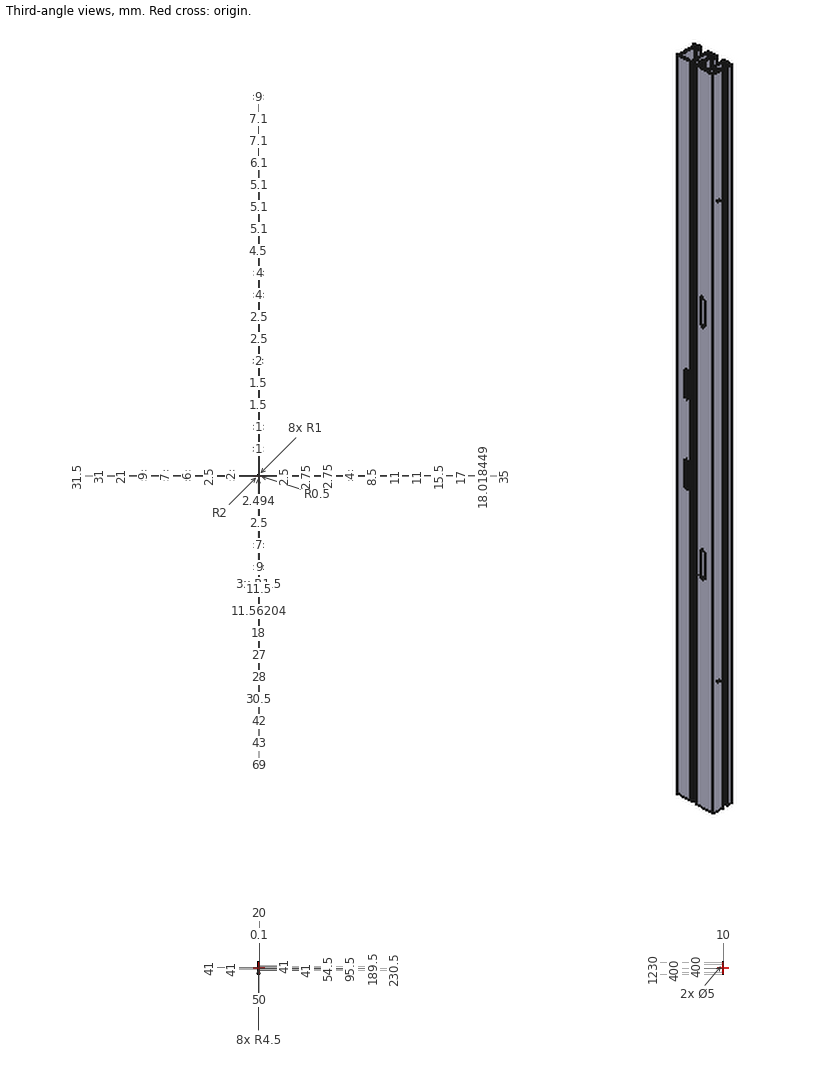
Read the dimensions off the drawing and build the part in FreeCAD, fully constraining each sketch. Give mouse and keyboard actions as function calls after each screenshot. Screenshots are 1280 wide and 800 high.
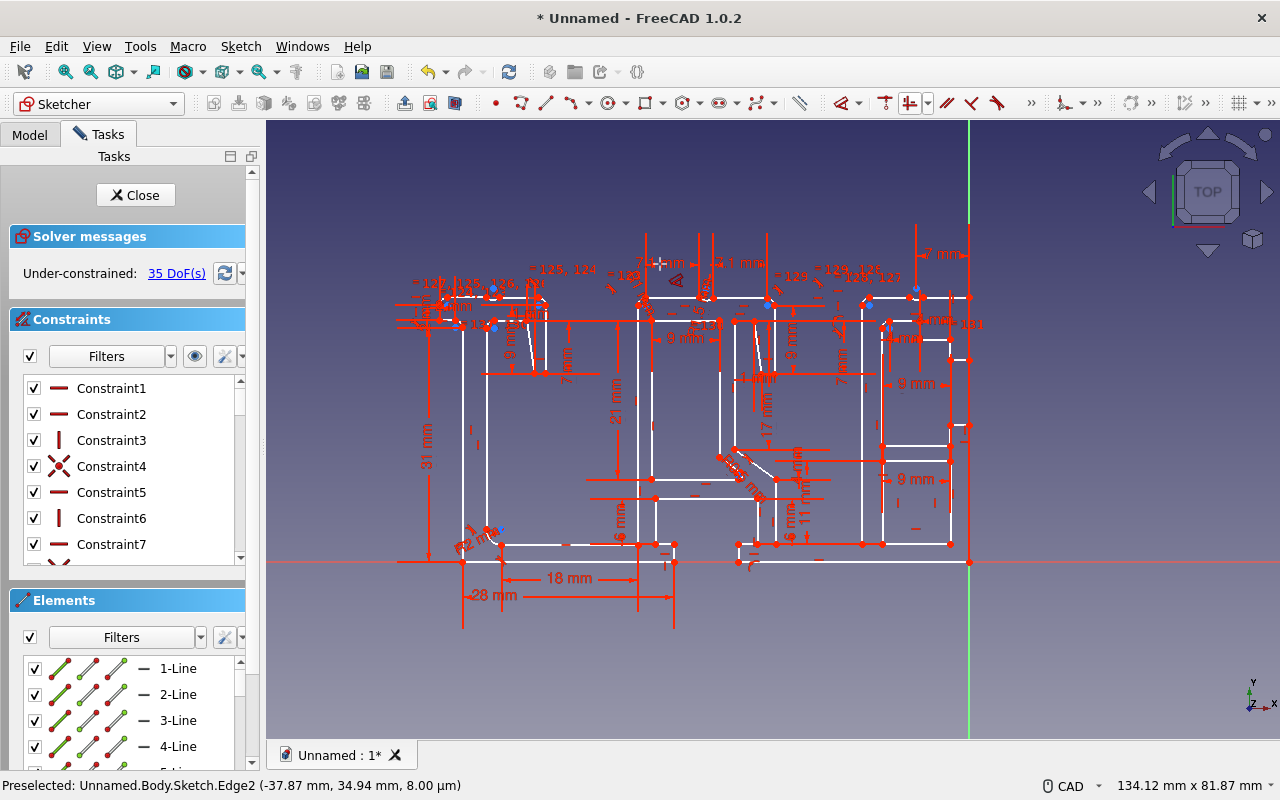
scroll(504, 321, up, 2)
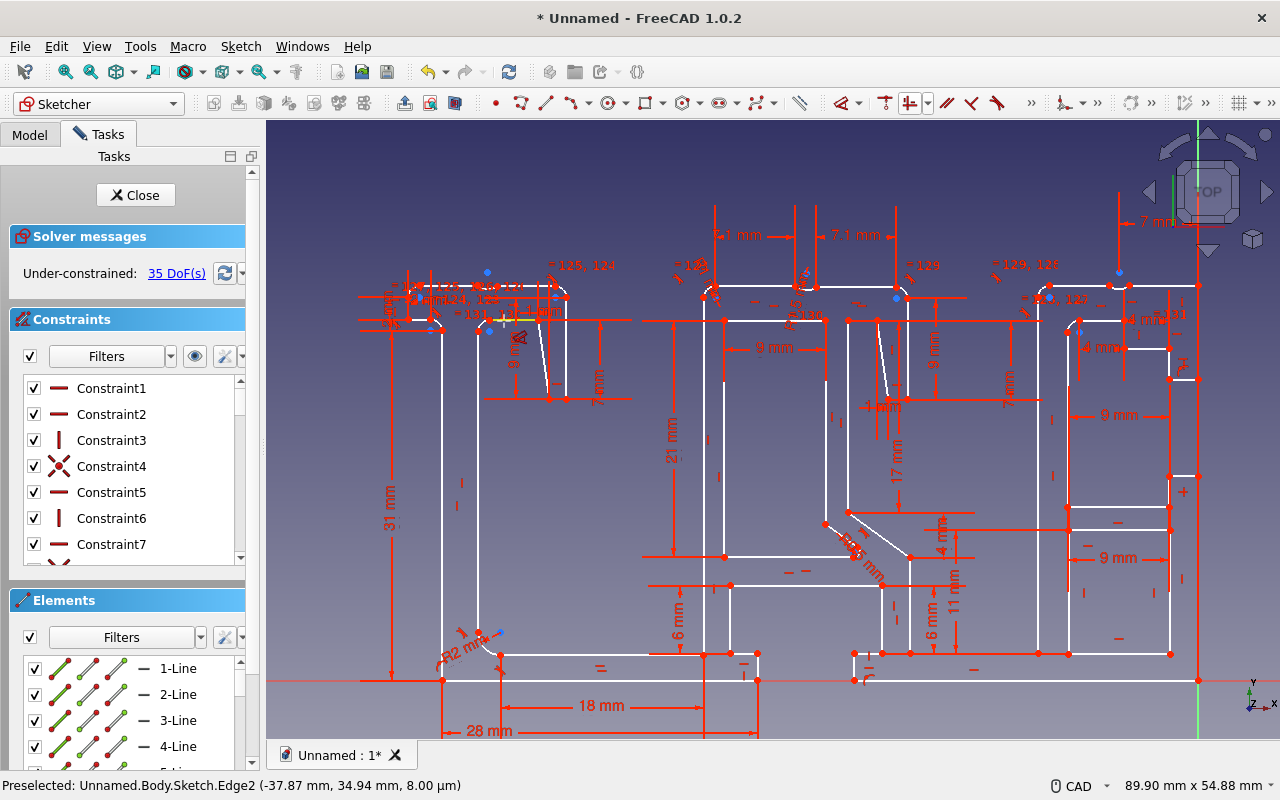
click(504, 320)
click(514, 262)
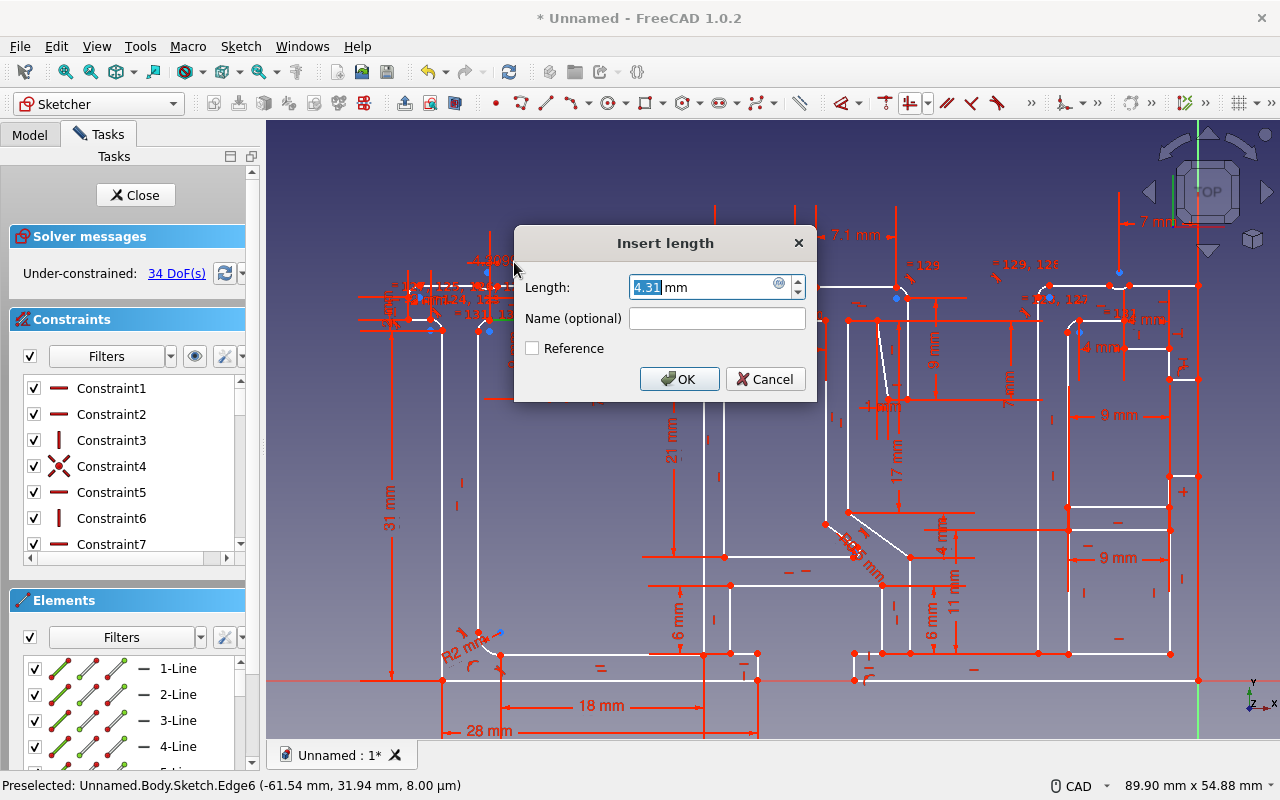
text(4.5)
key(Return)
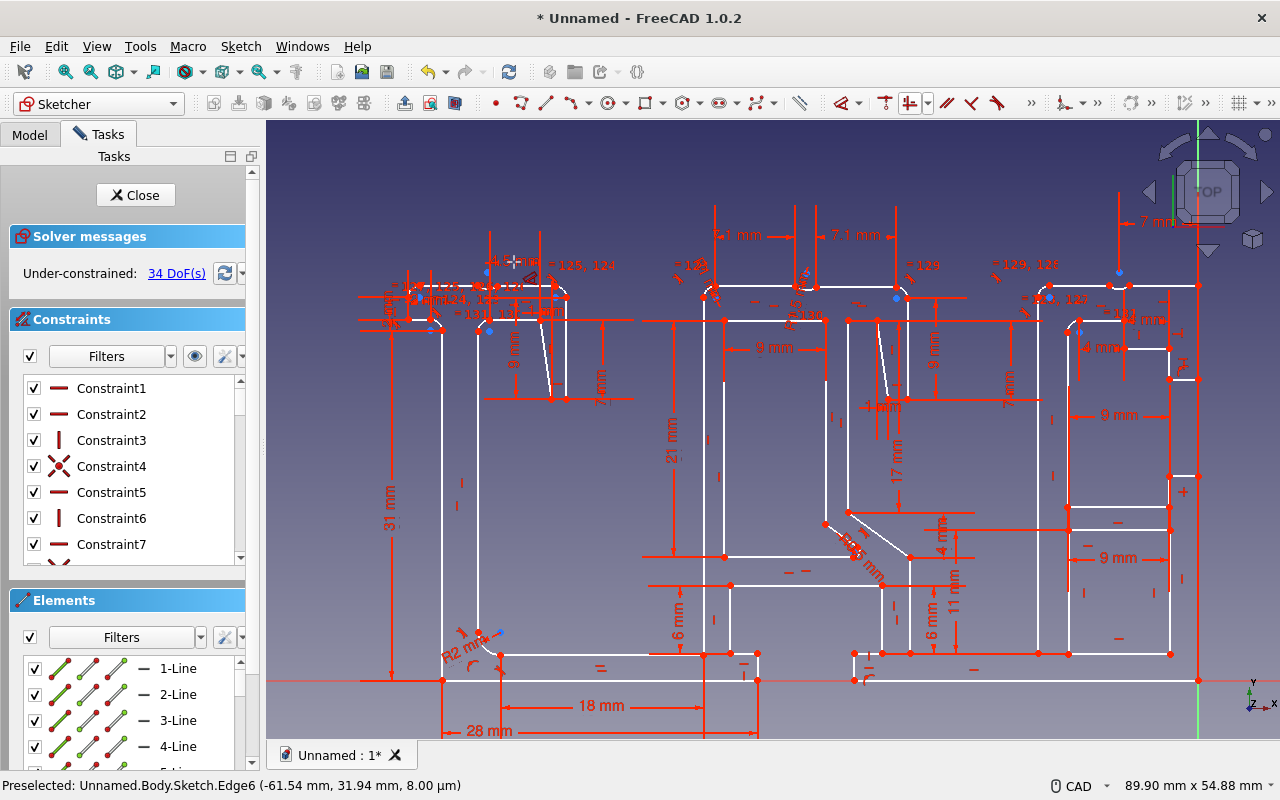
scroll(559, 399, up, 5)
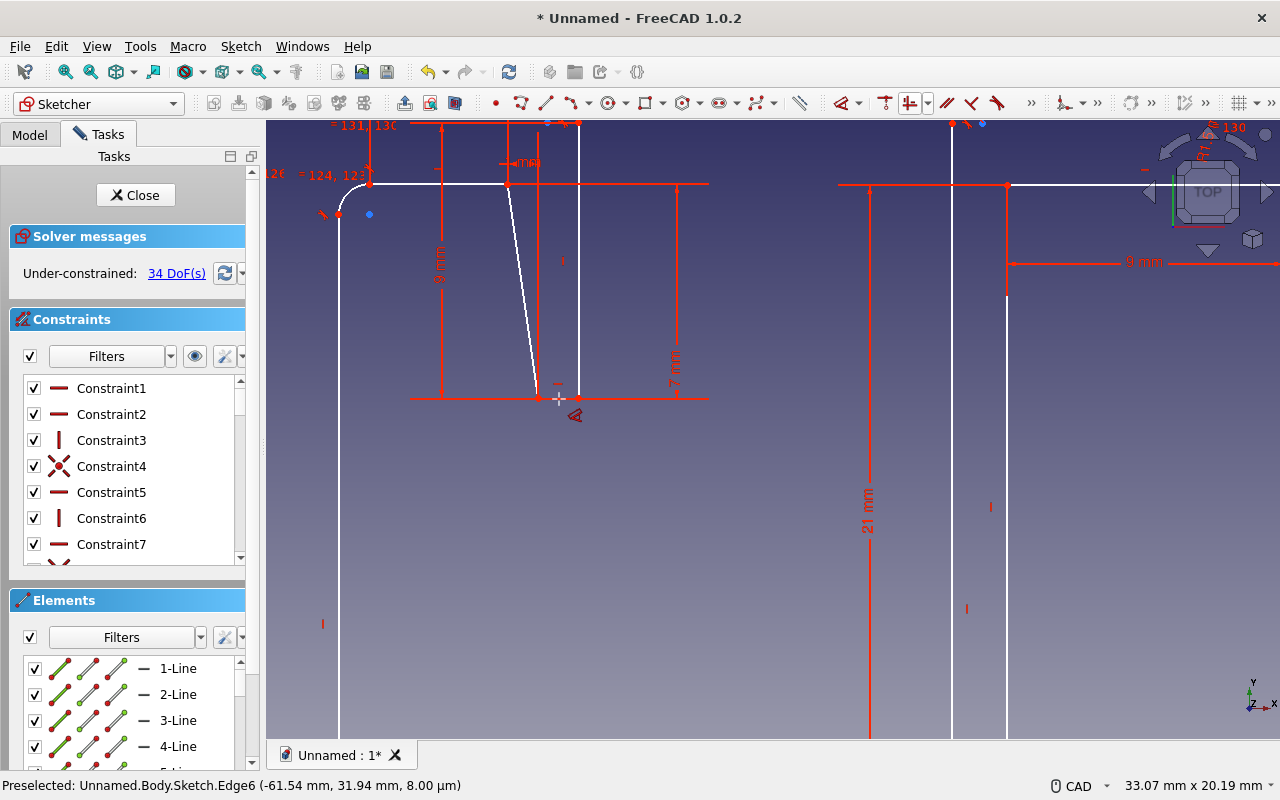
click(558, 399)
click(558, 365)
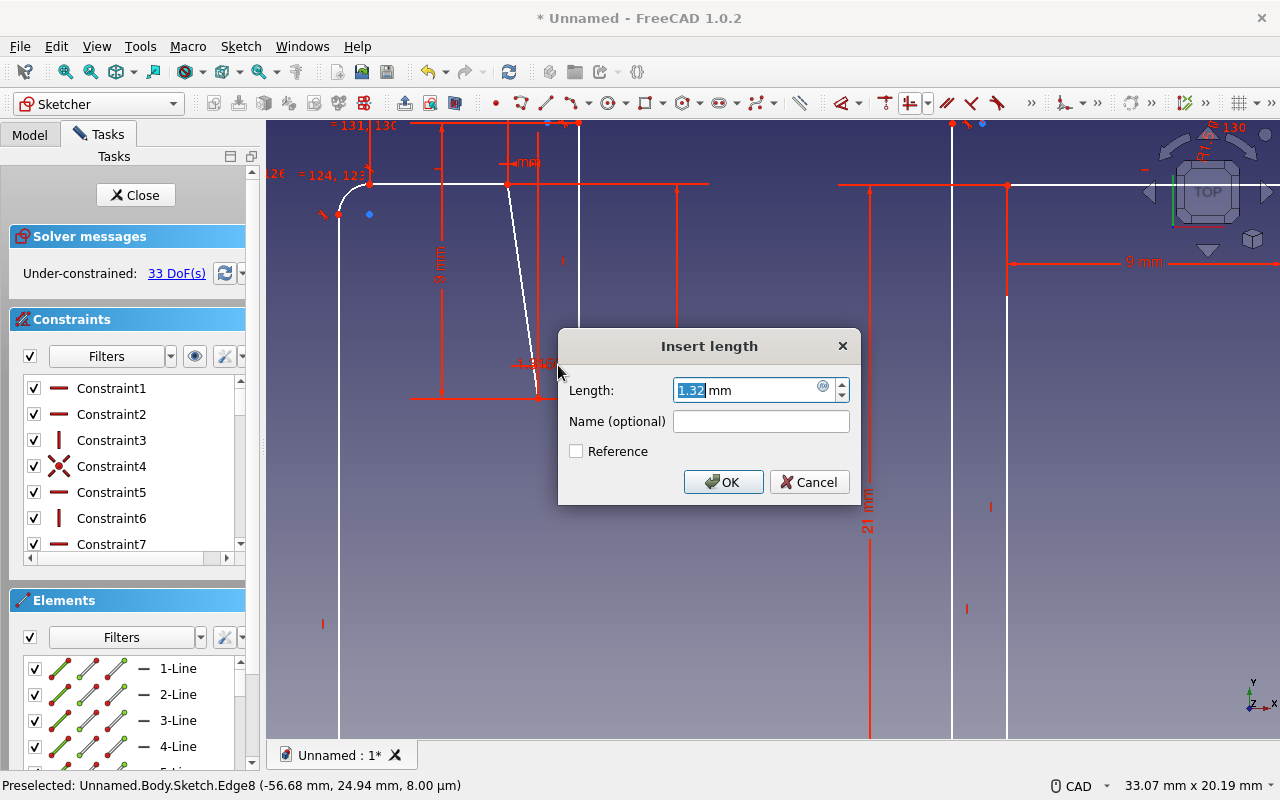
text(1.5)
key(Return)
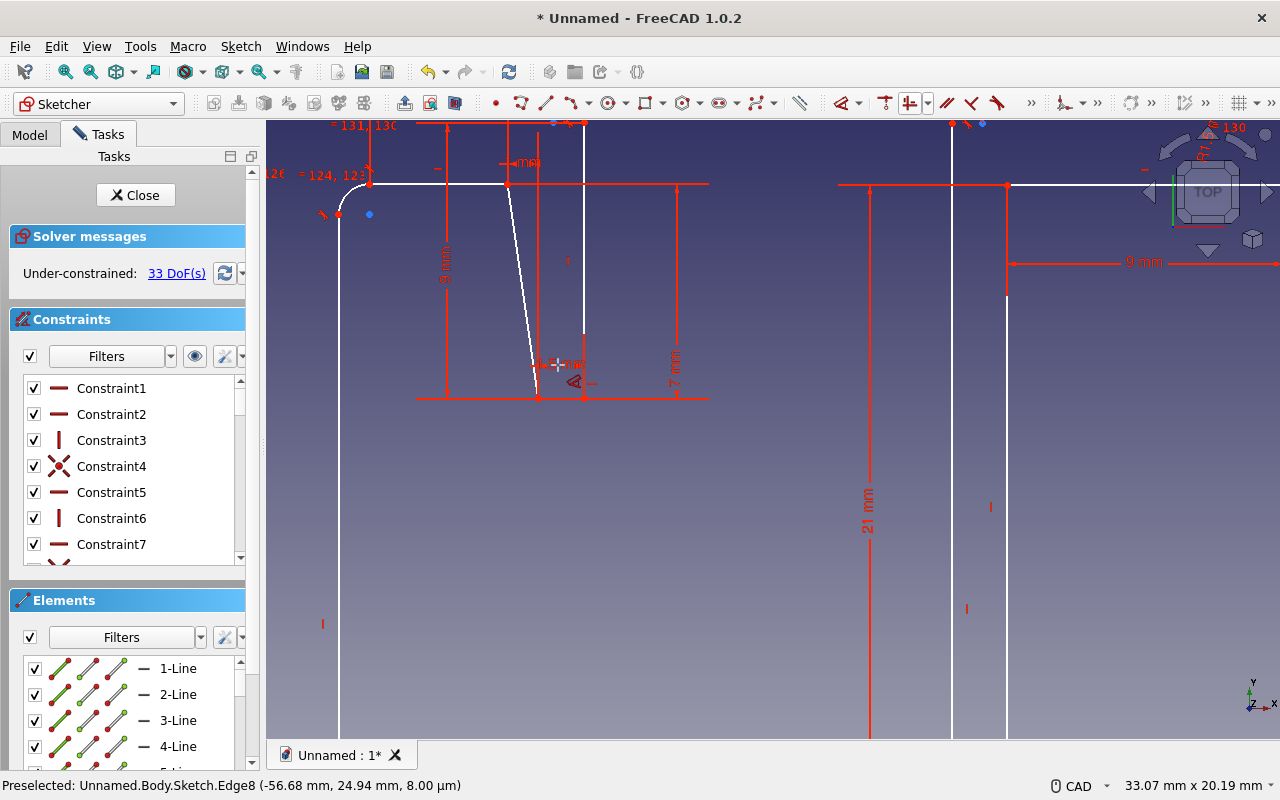
scroll(535, 365, down, 7)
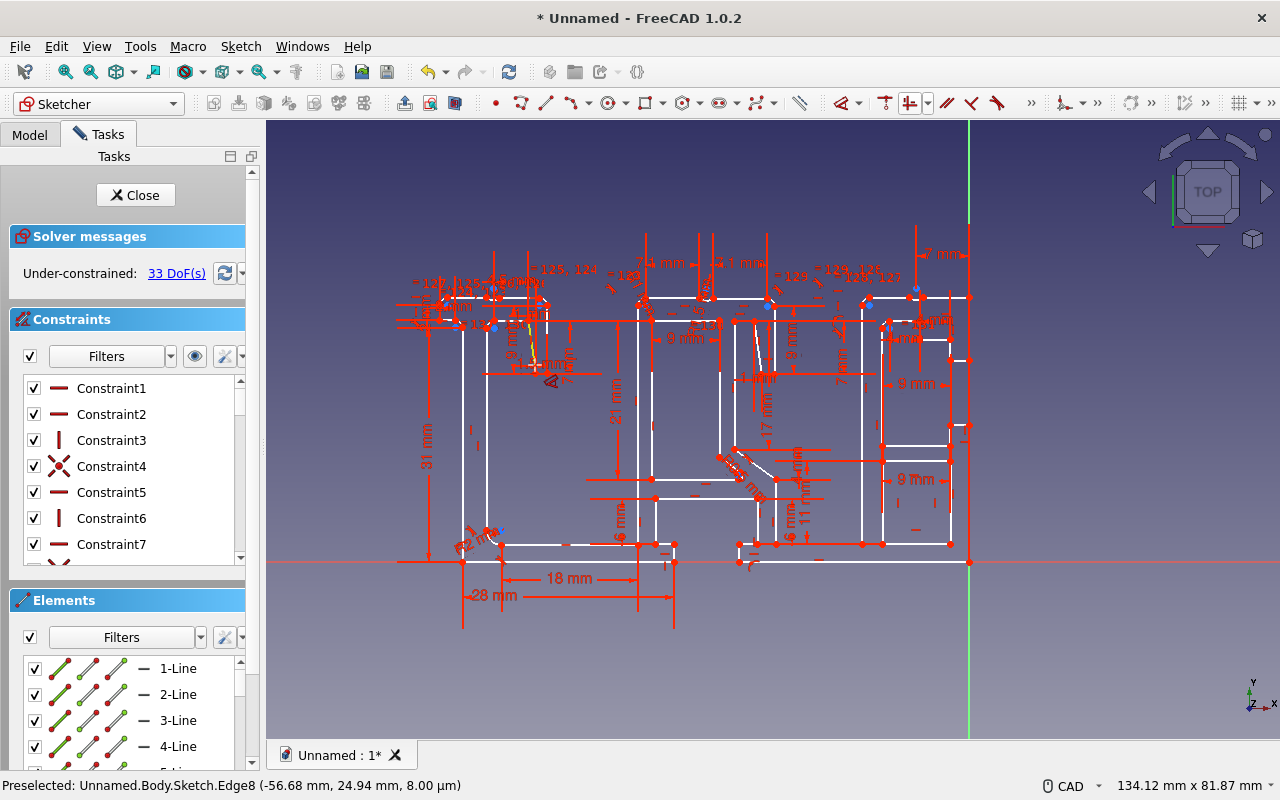
click(528, 298)
click(520, 240)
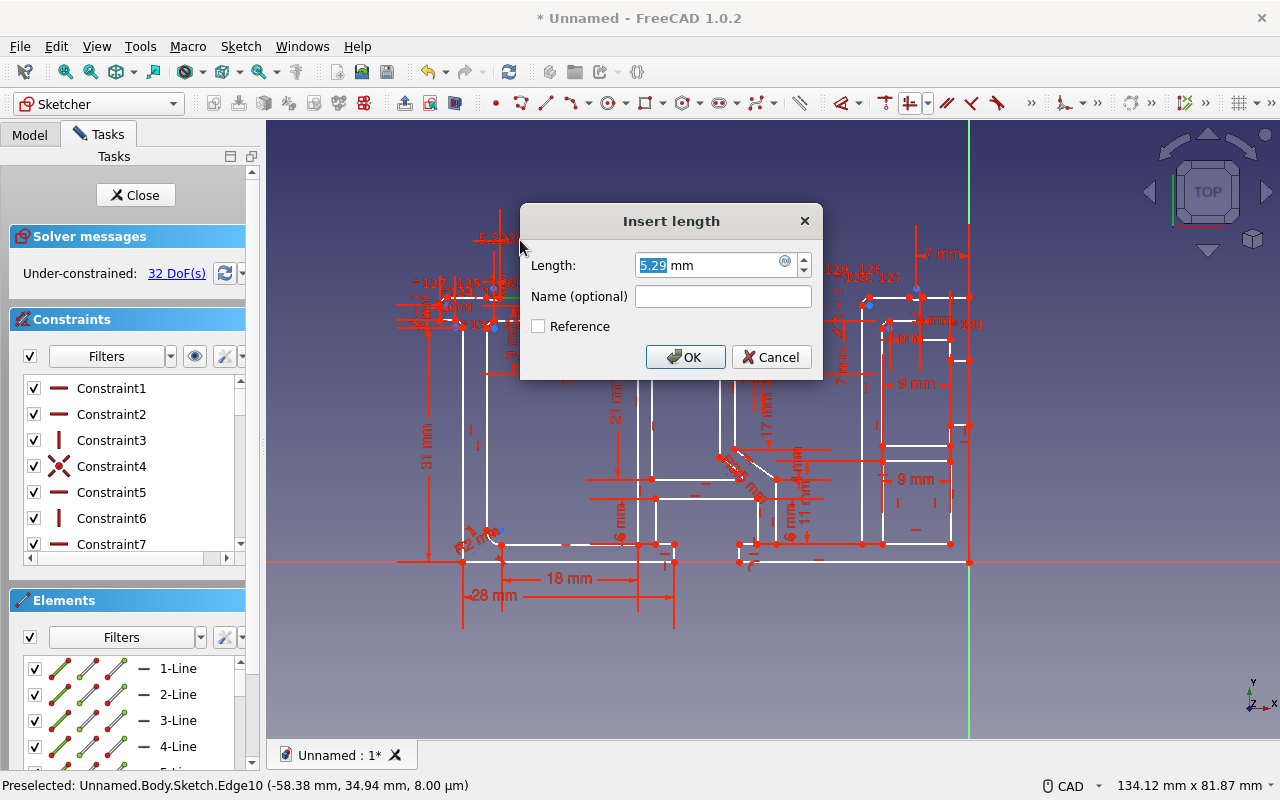
text(5.1)
key(Return)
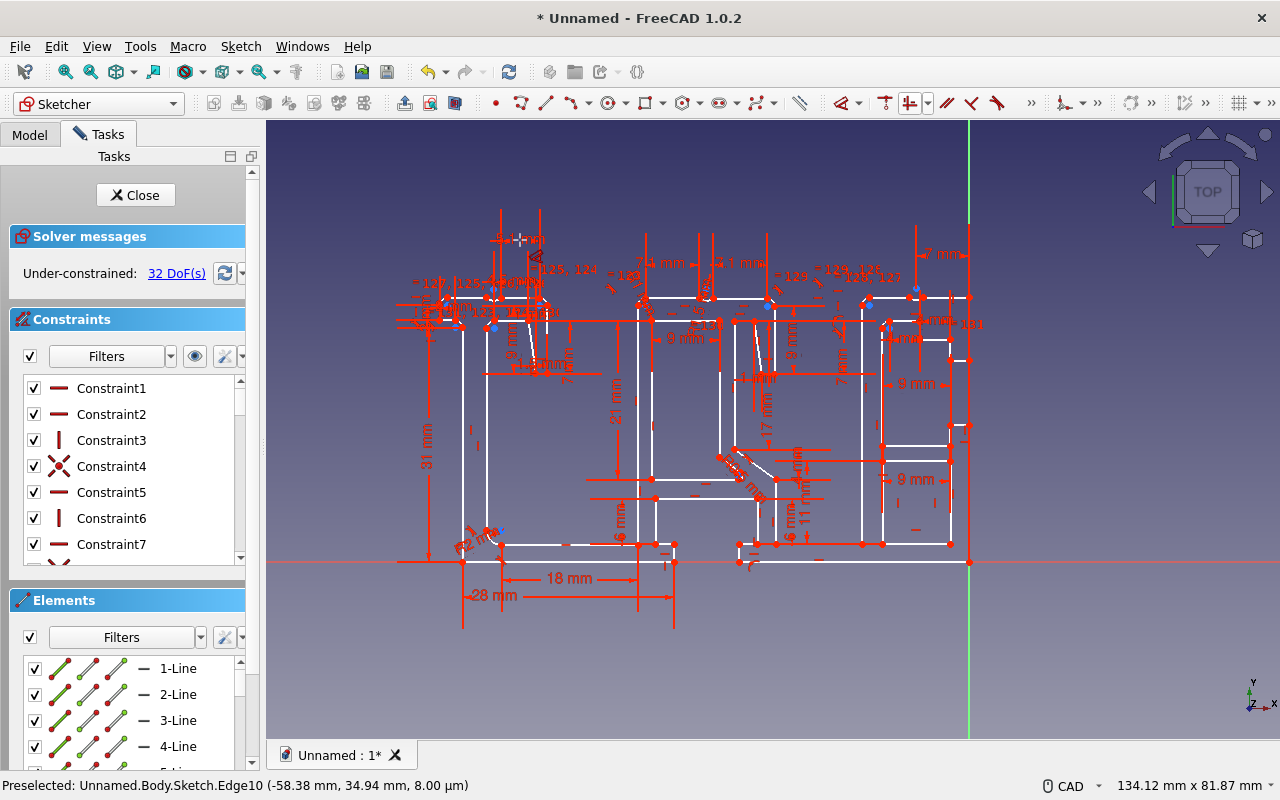
click(475, 298)
click(467, 216)